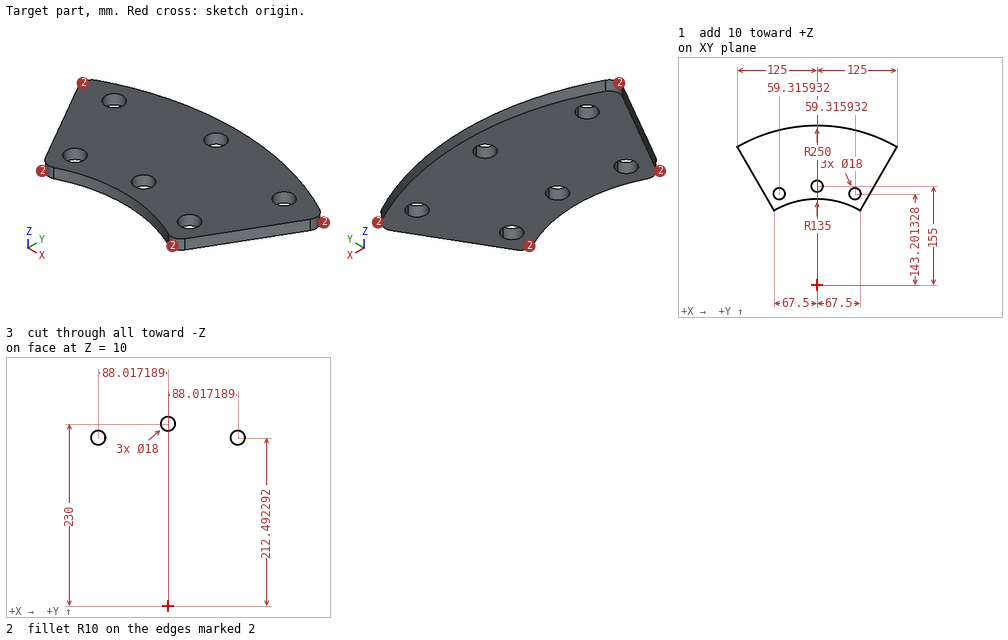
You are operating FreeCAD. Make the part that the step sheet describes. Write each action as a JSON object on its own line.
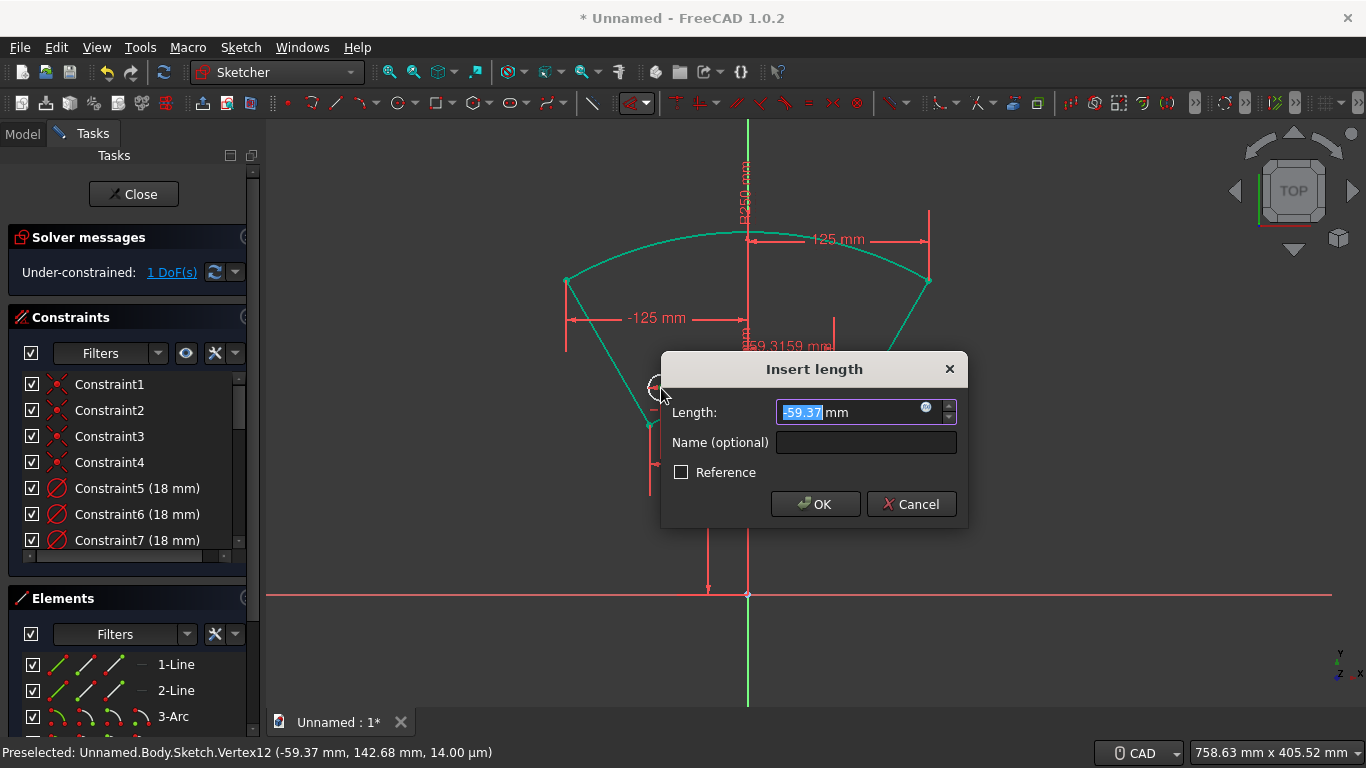
{"action": "type", "text": "-59.315932"}
{"action": "key", "text": "Return"}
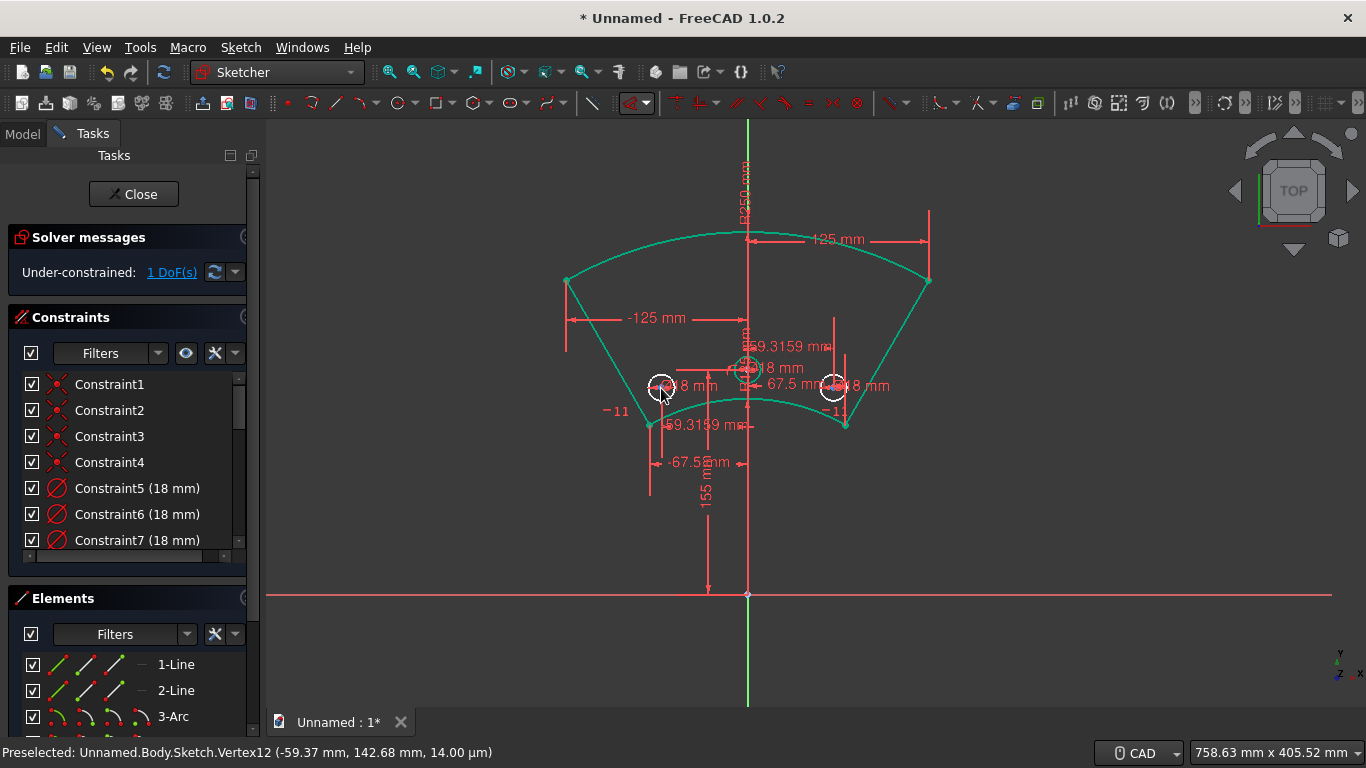
{"action": "left_click", "coordinate": [834, 388]}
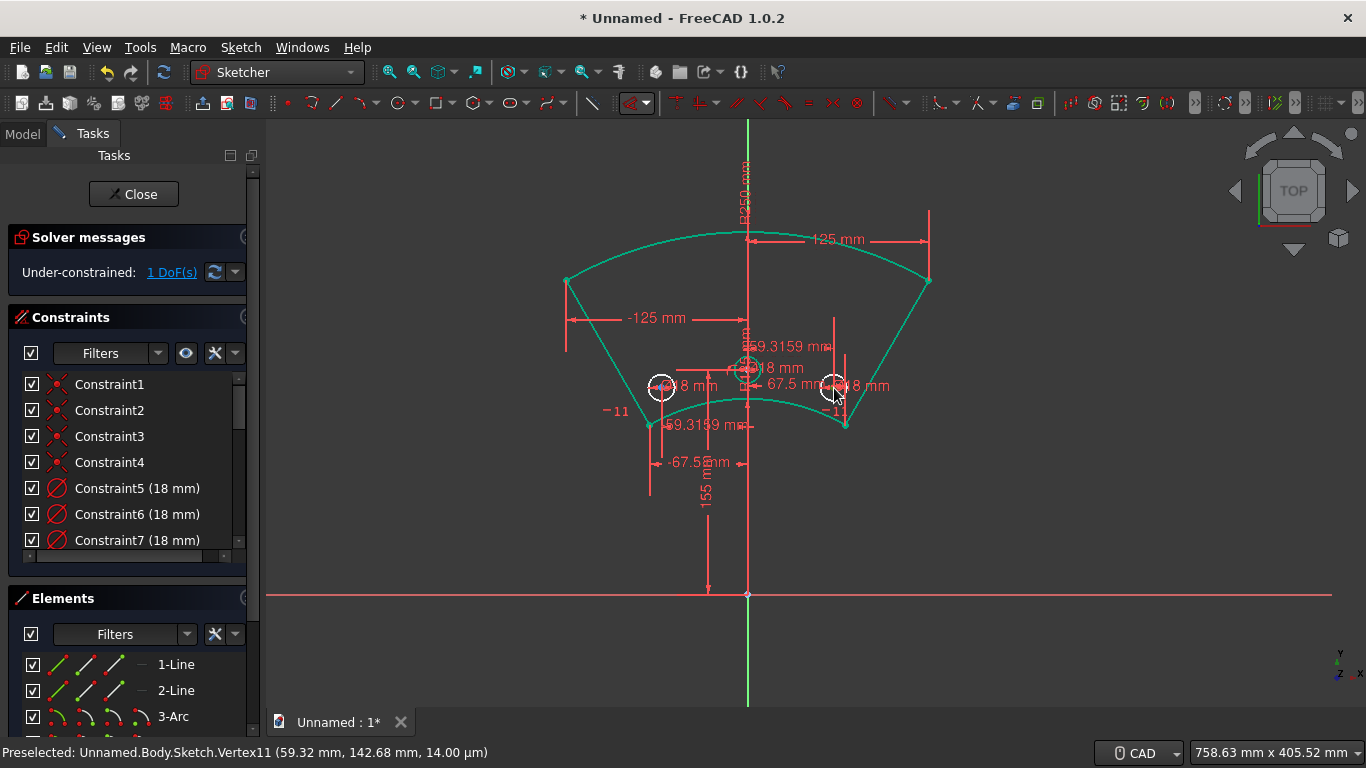
{"action": "left_click", "coordinate": [648, 104]}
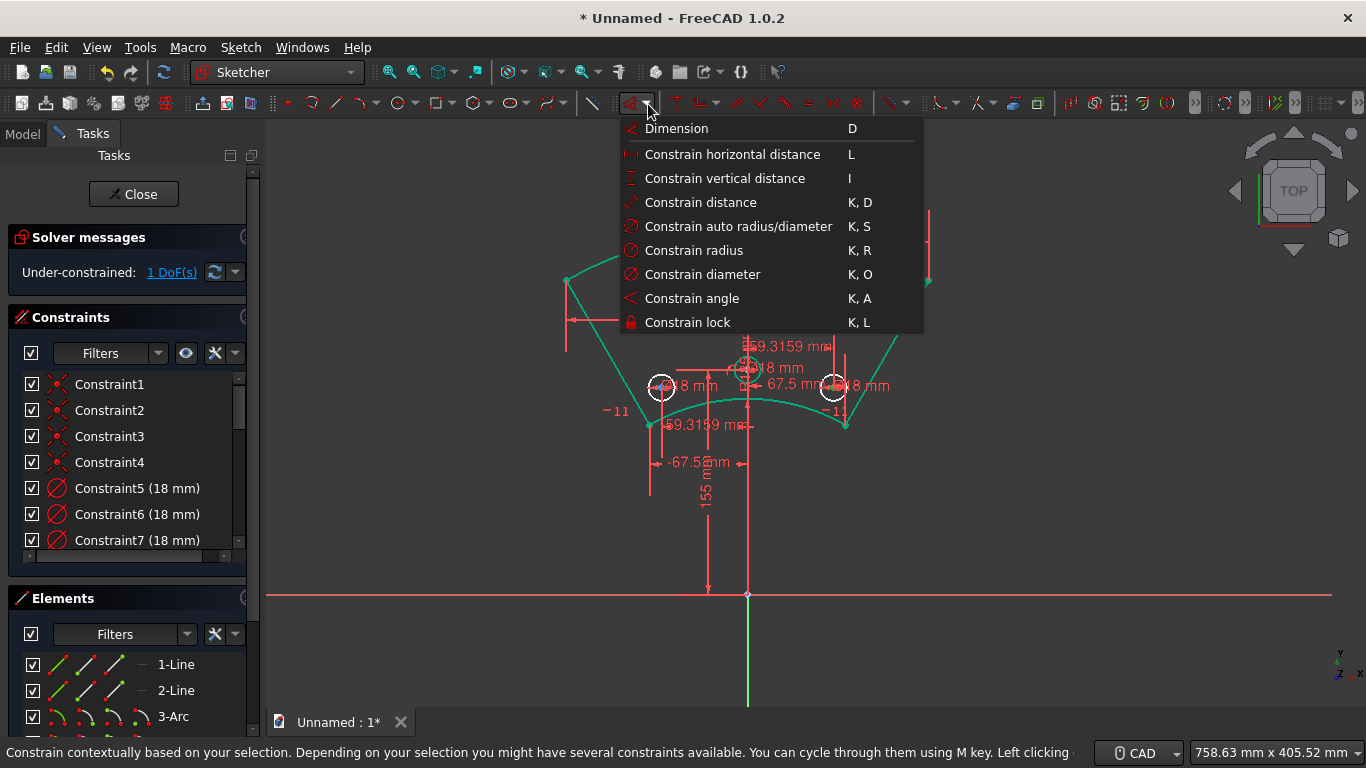
{"action": "left_click", "coordinate": [772, 178]}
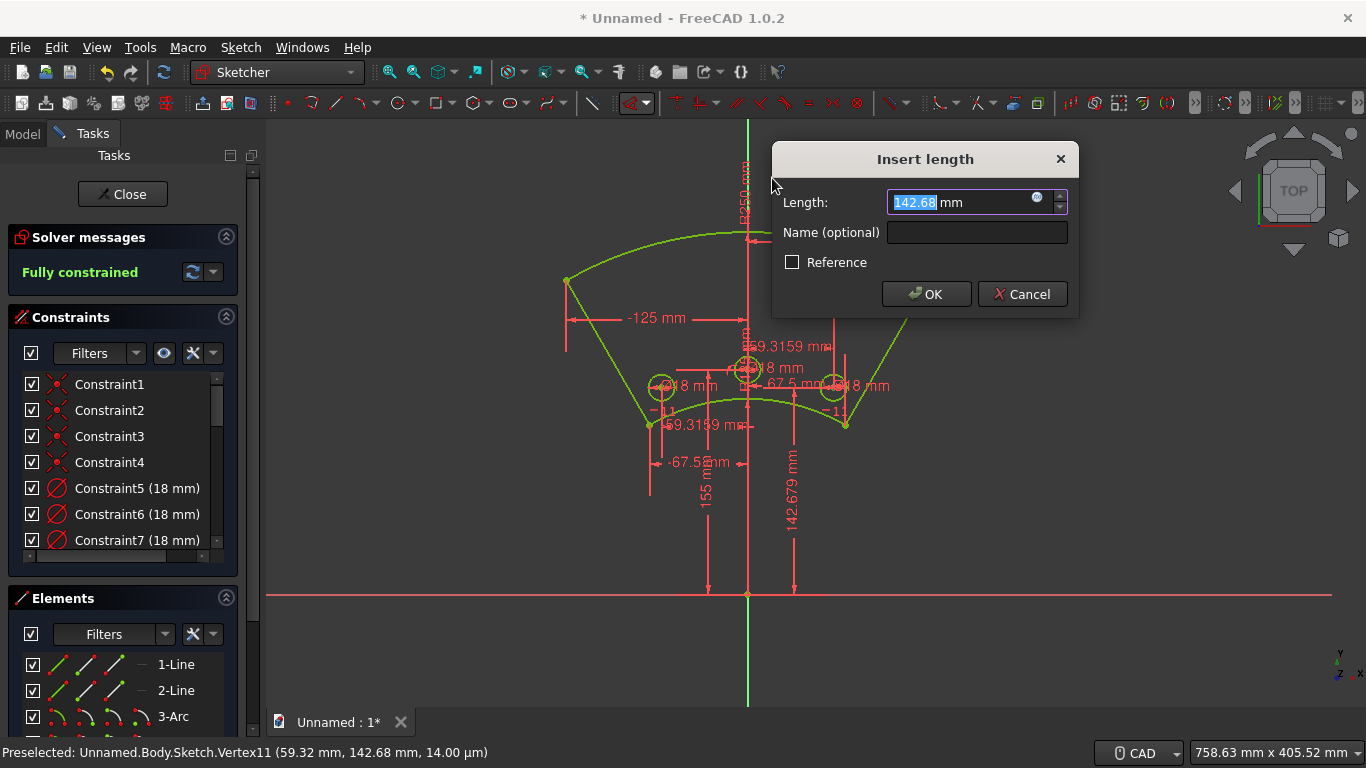
{"action": "type", "text": "143.201328"}
{"action": "key", "text": "Return"}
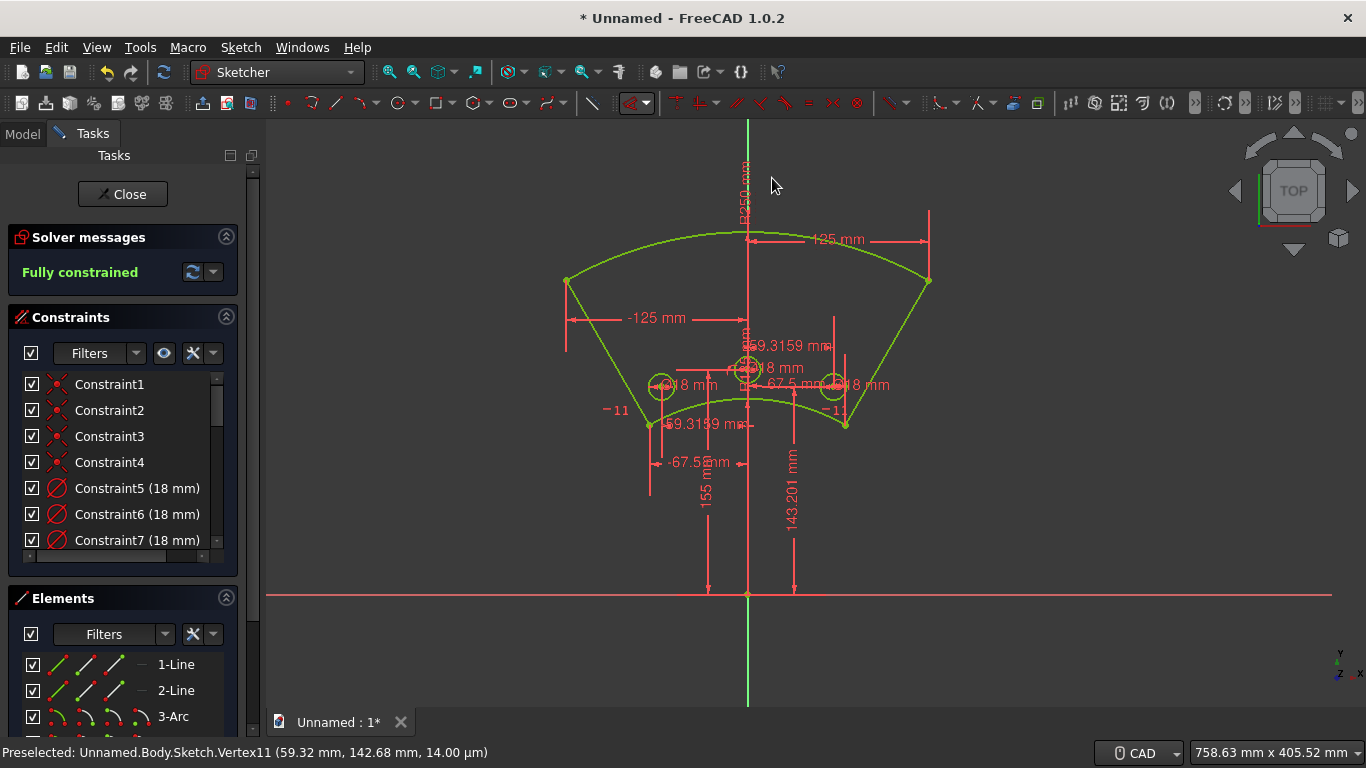
{"action": "left_click", "coordinate": [123, 194]}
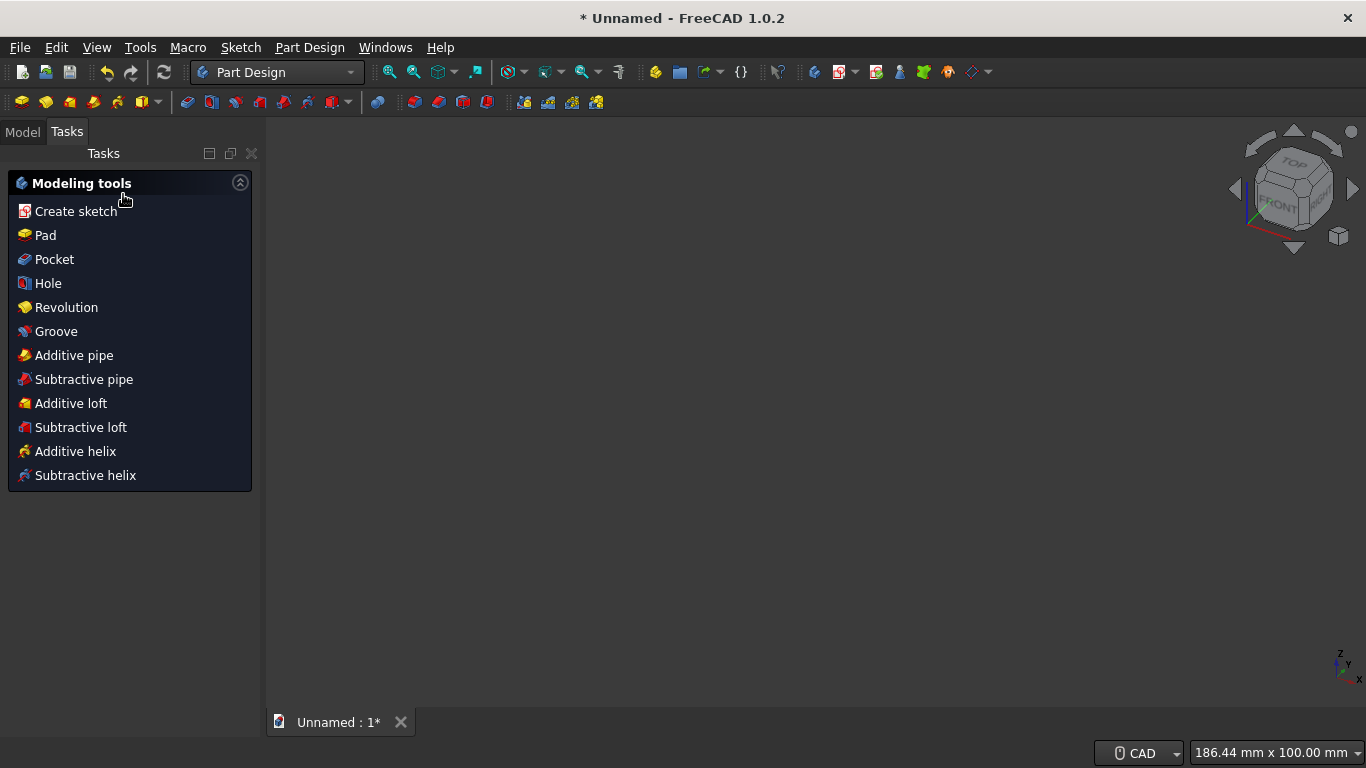
{"action": "left_click", "coordinate": [22, 102]}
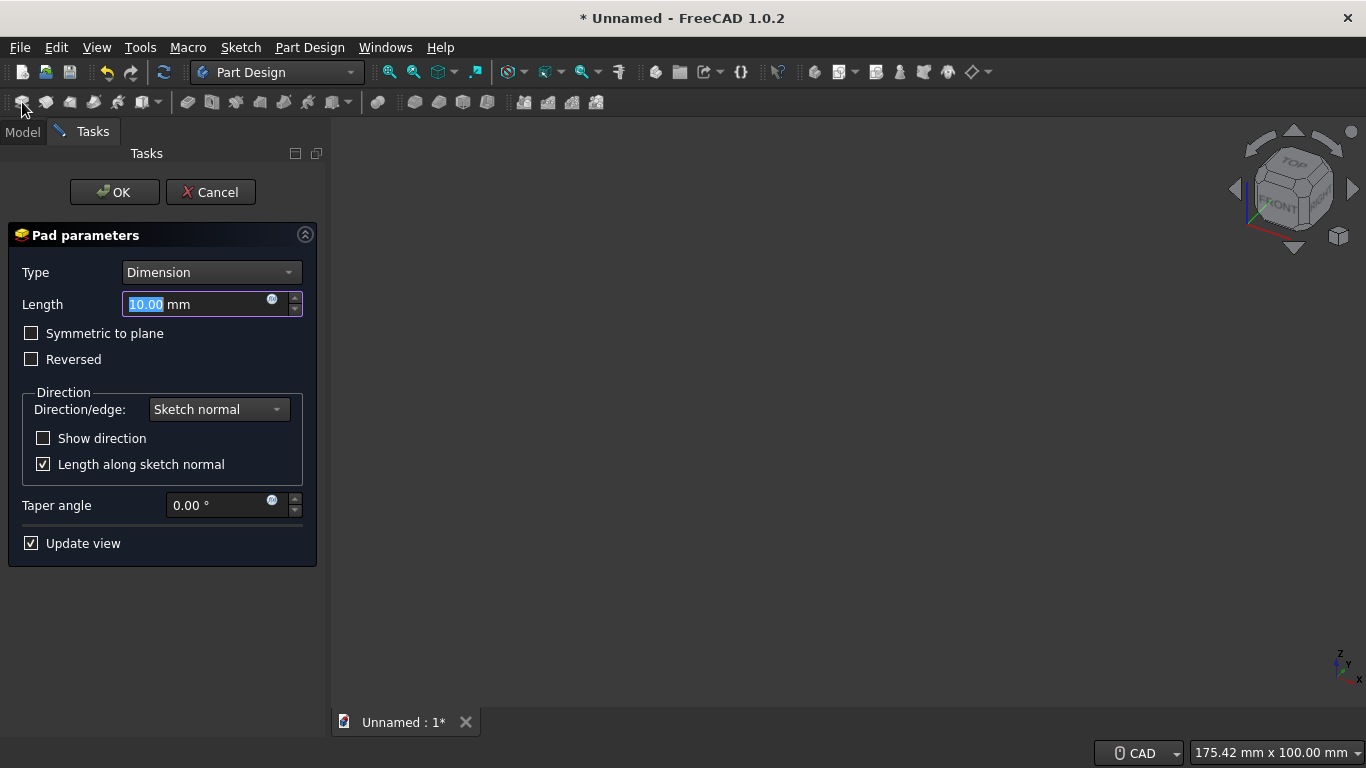
{"action": "type", "text": "10"}
{"action": "key", "text": "Tab"}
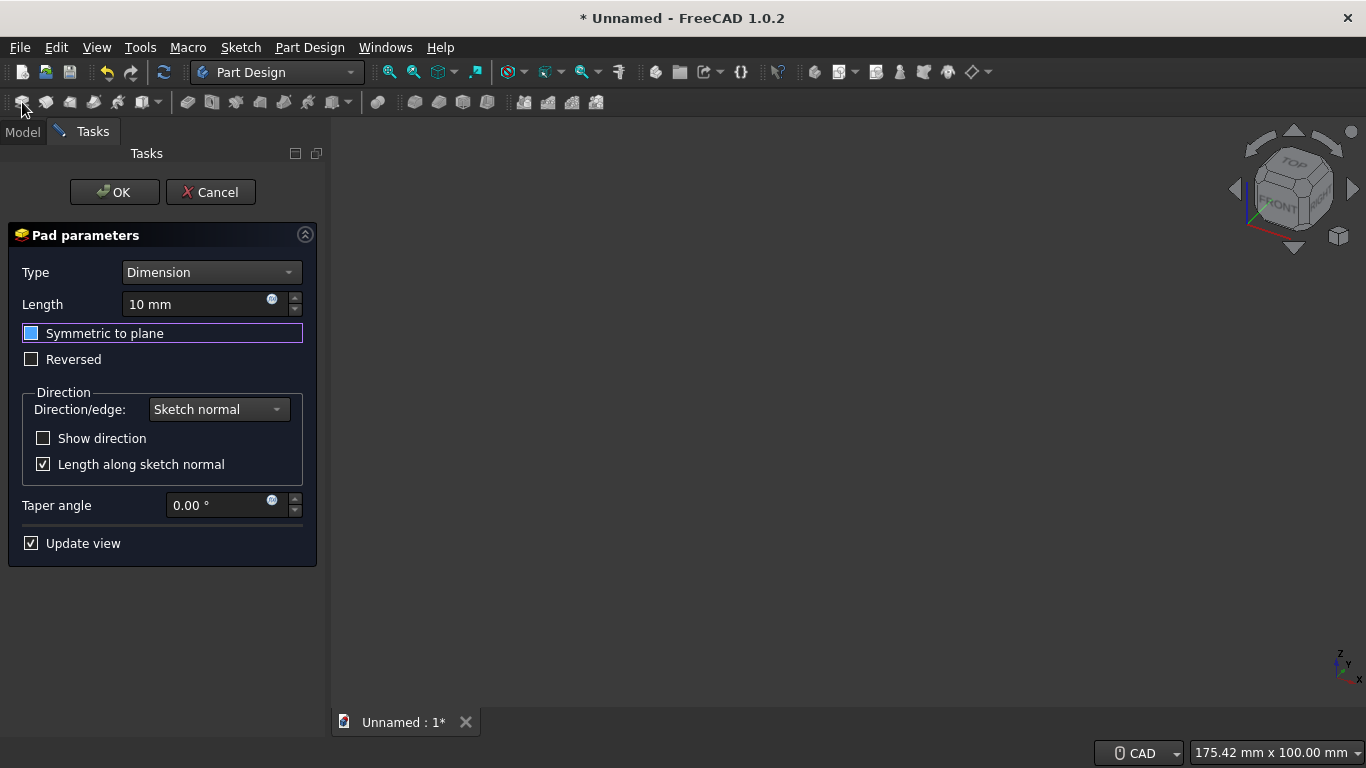
{"action": "left_click", "coordinate": [115, 192]}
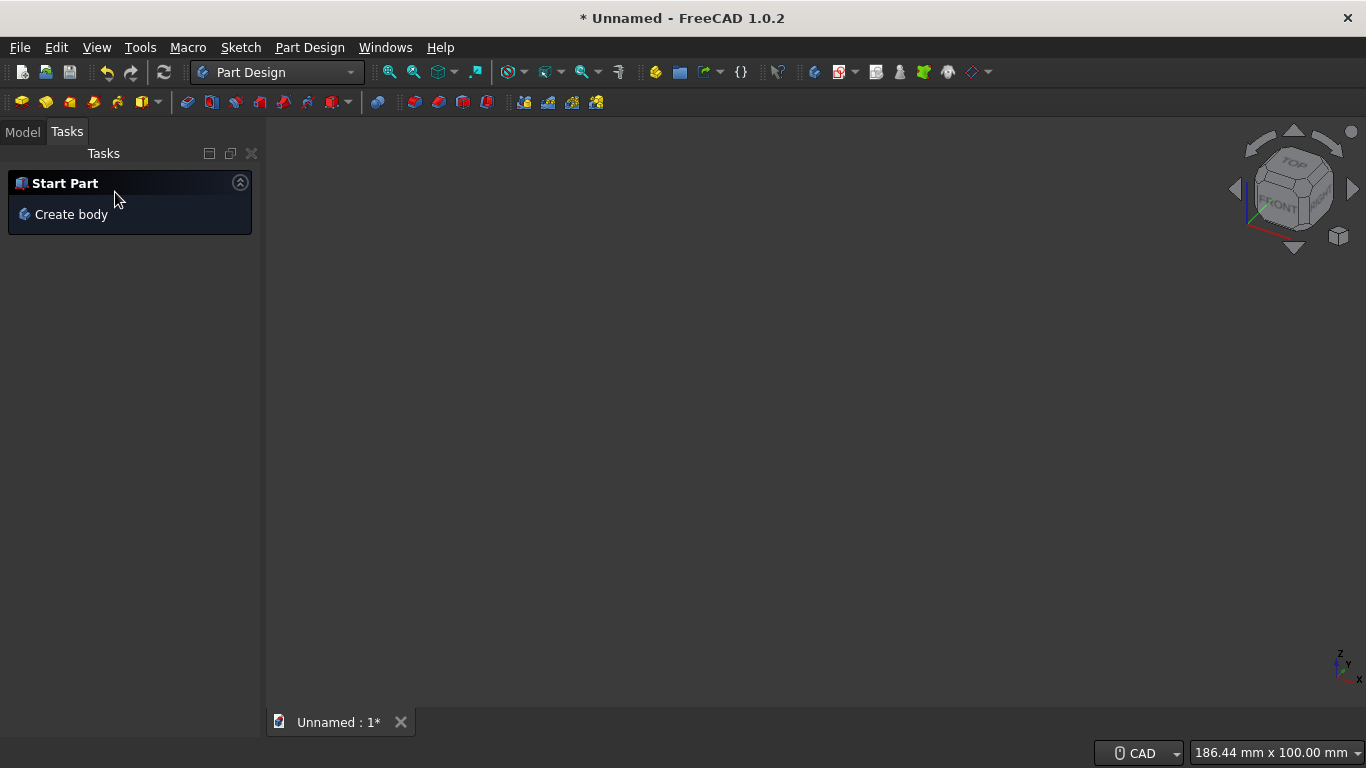
{"action": "left_click", "coordinate": [390, 72]}